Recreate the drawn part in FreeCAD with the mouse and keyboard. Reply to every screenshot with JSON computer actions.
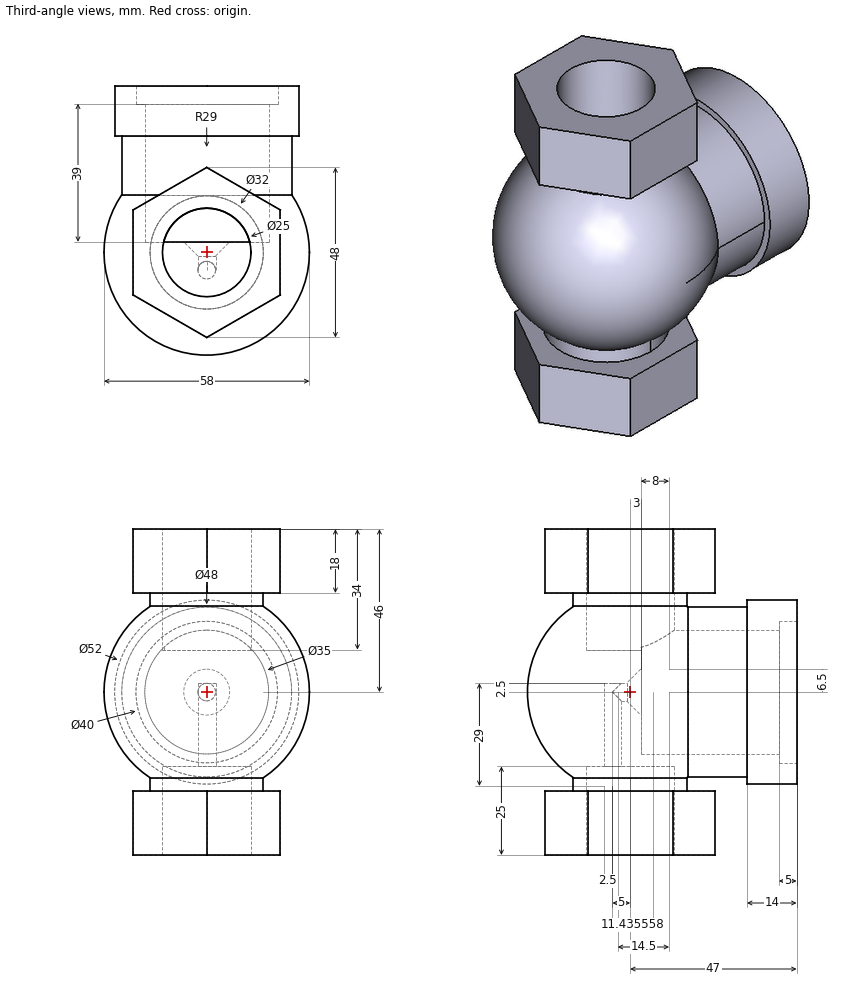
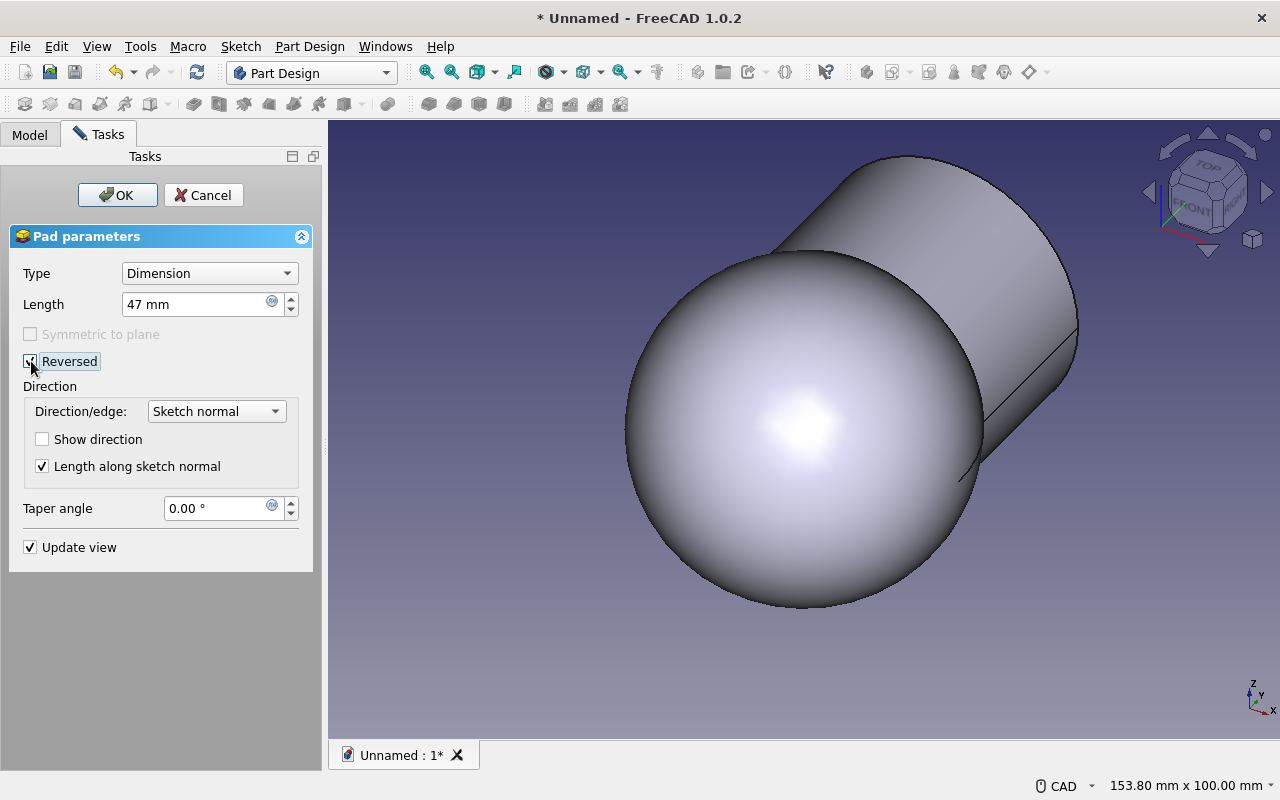
{"action": "left_click", "coordinate": [118, 195]}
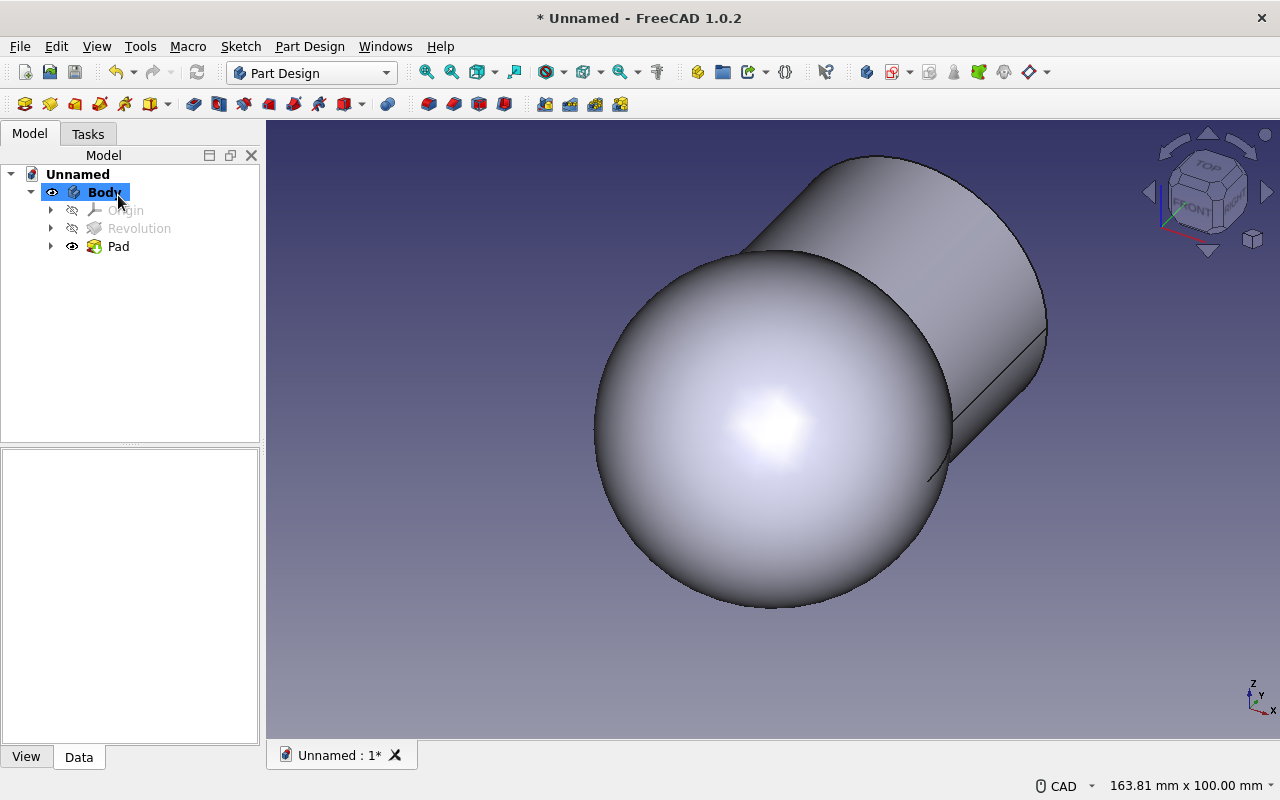
{"action": "left_click", "coordinate": [427, 72]}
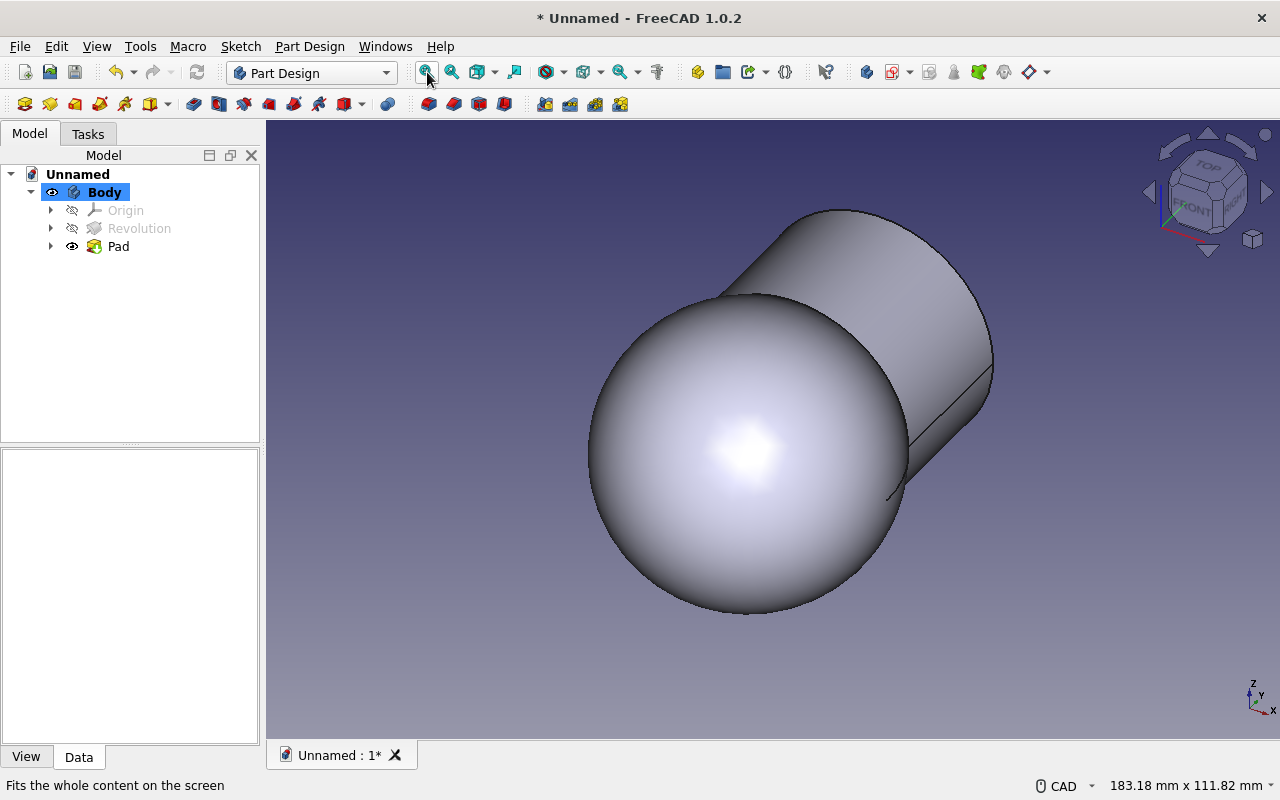
{"action": "key", "text": "4"}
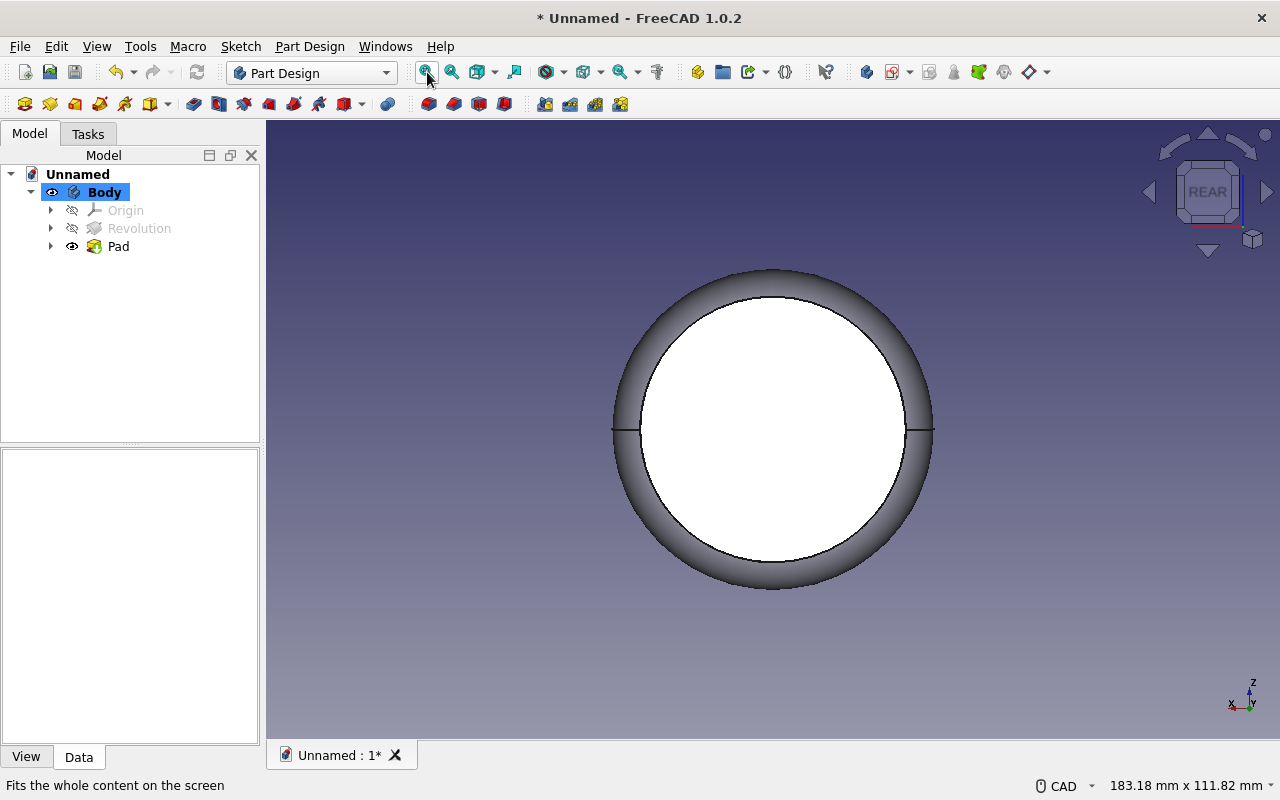
{"action": "left_click", "coordinate": [773, 429]}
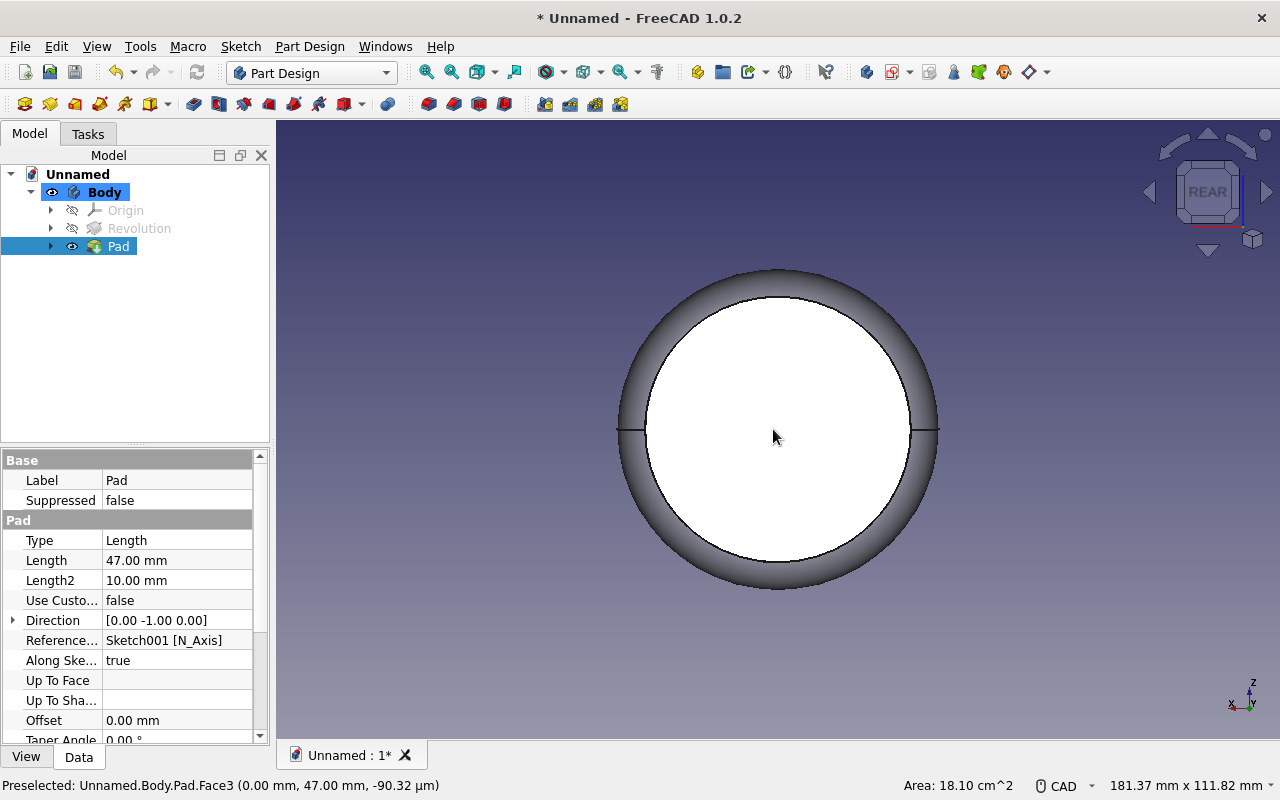
{"action": "left_click", "coordinate": [892, 72]}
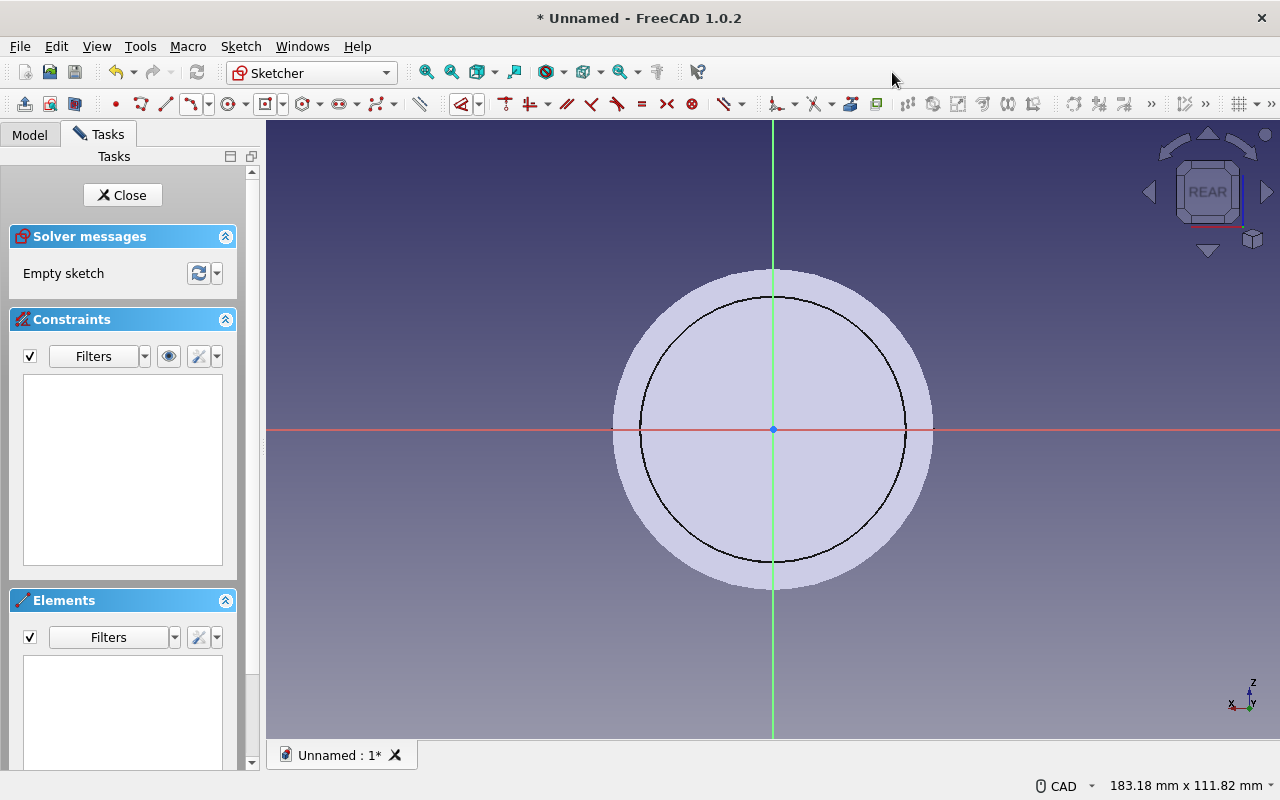
{"action": "scroll", "coordinate": [912, 430], "scroll_direction": "up", "scroll_amount": 2}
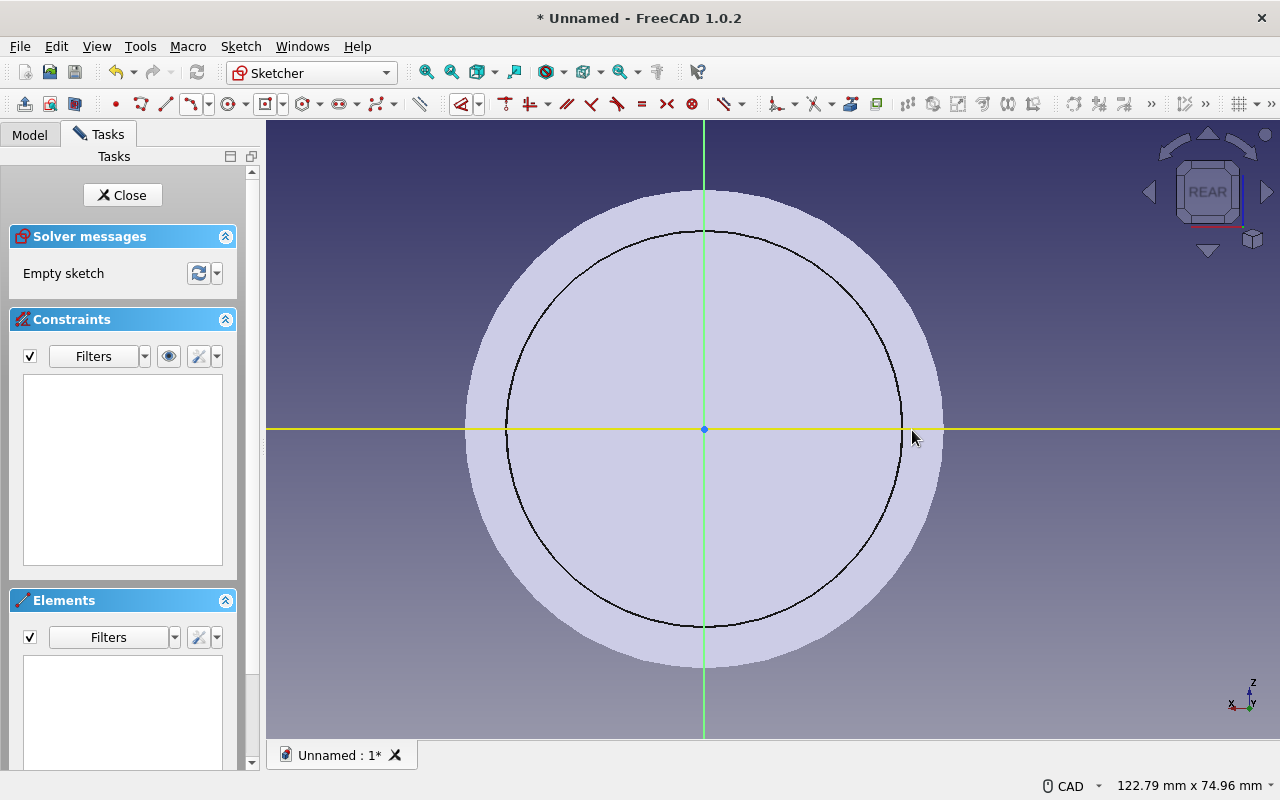
{"action": "left_click", "coordinate": [228, 104]}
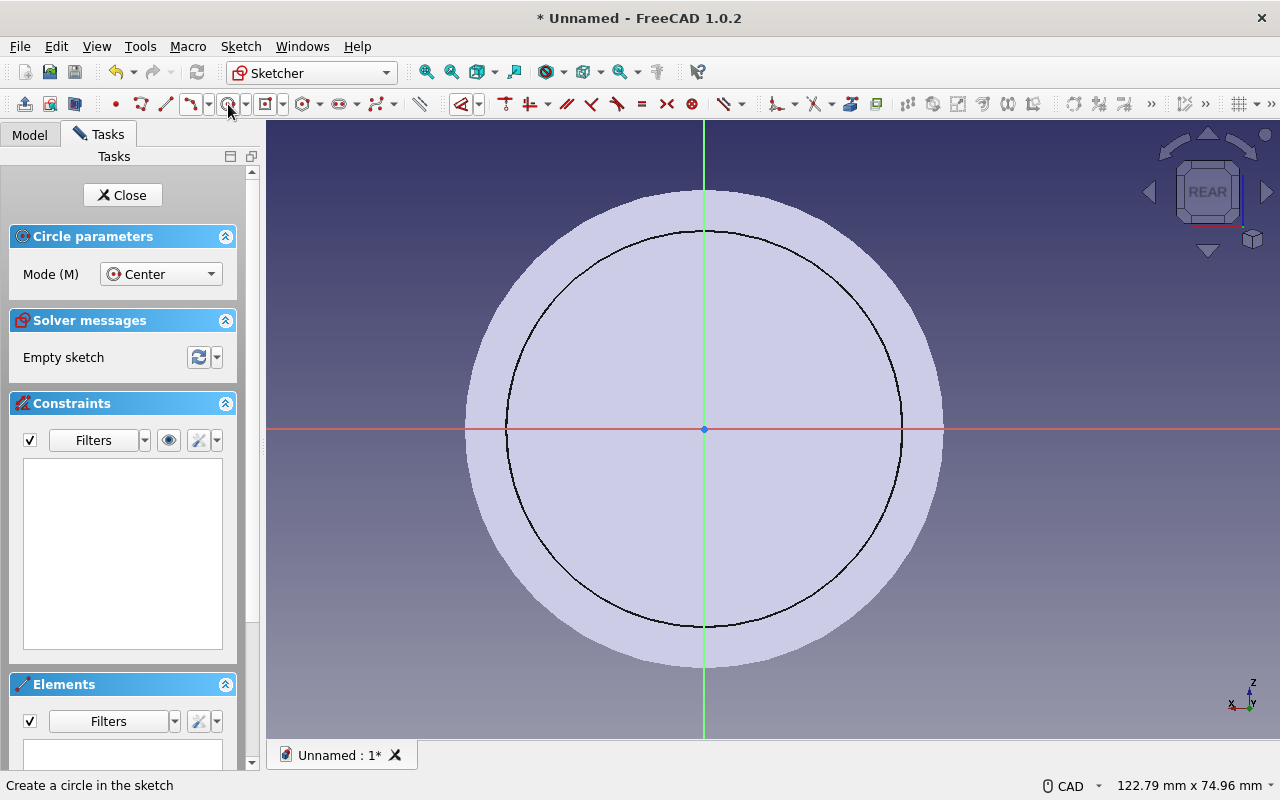
{"action": "left_click", "coordinate": [704, 429]}
{"action": "left_click", "coordinate": [856, 277]}
{"action": "key", "text": "Escape"}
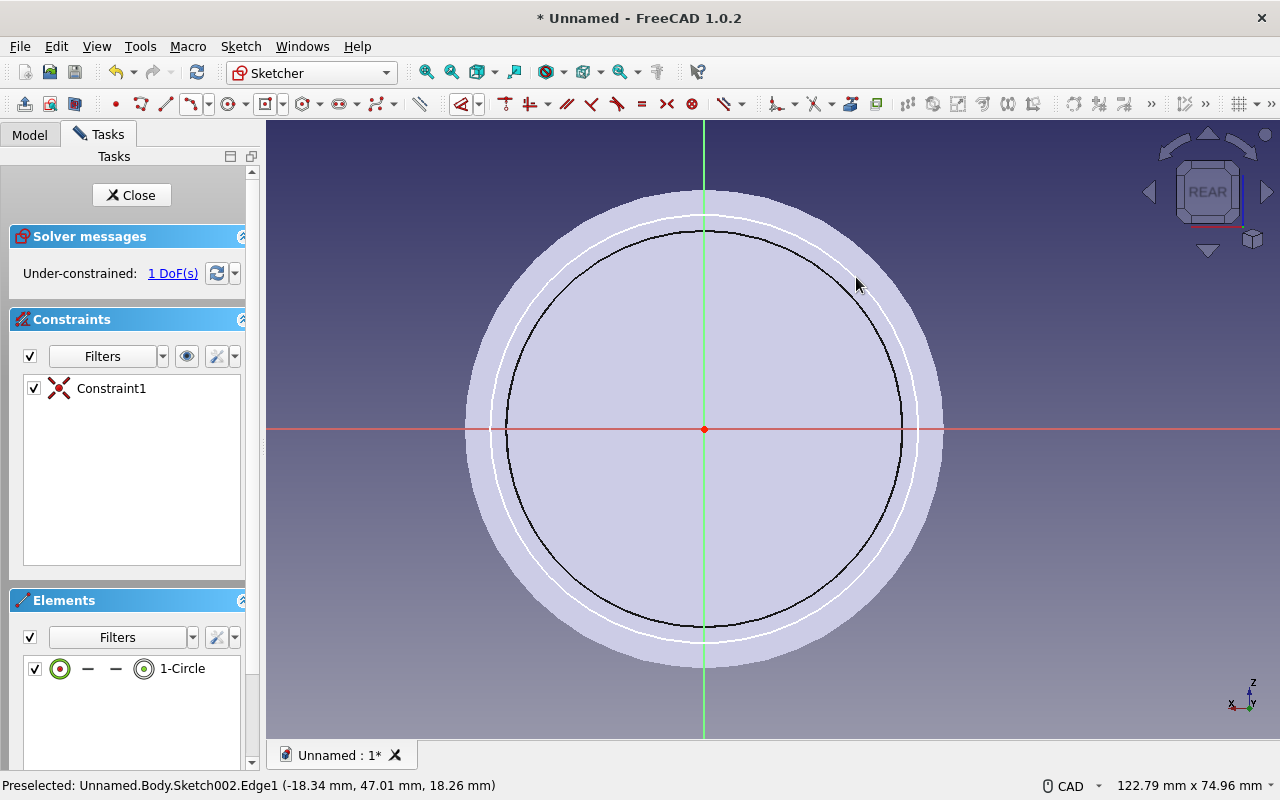
{"action": "left_click", "coordinate": [855, 277]}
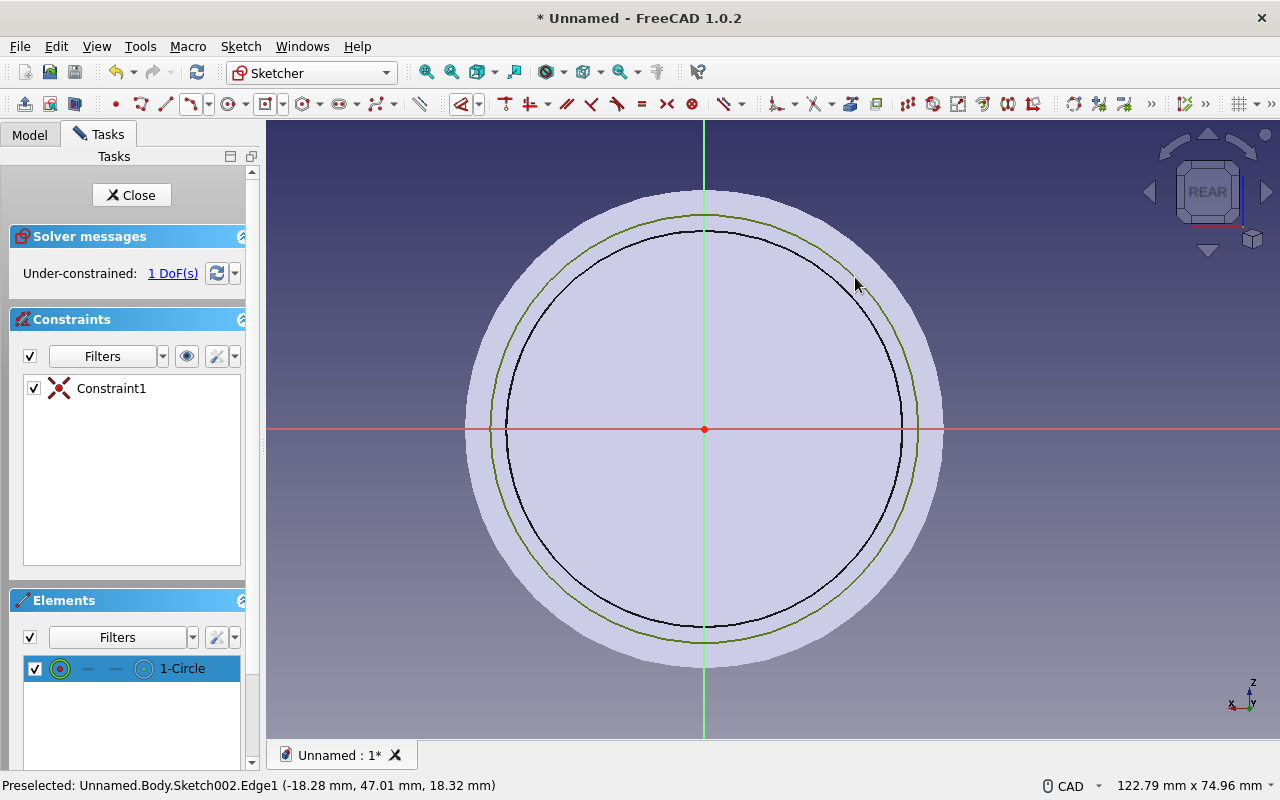
{"action": "key", "text": "k o"}